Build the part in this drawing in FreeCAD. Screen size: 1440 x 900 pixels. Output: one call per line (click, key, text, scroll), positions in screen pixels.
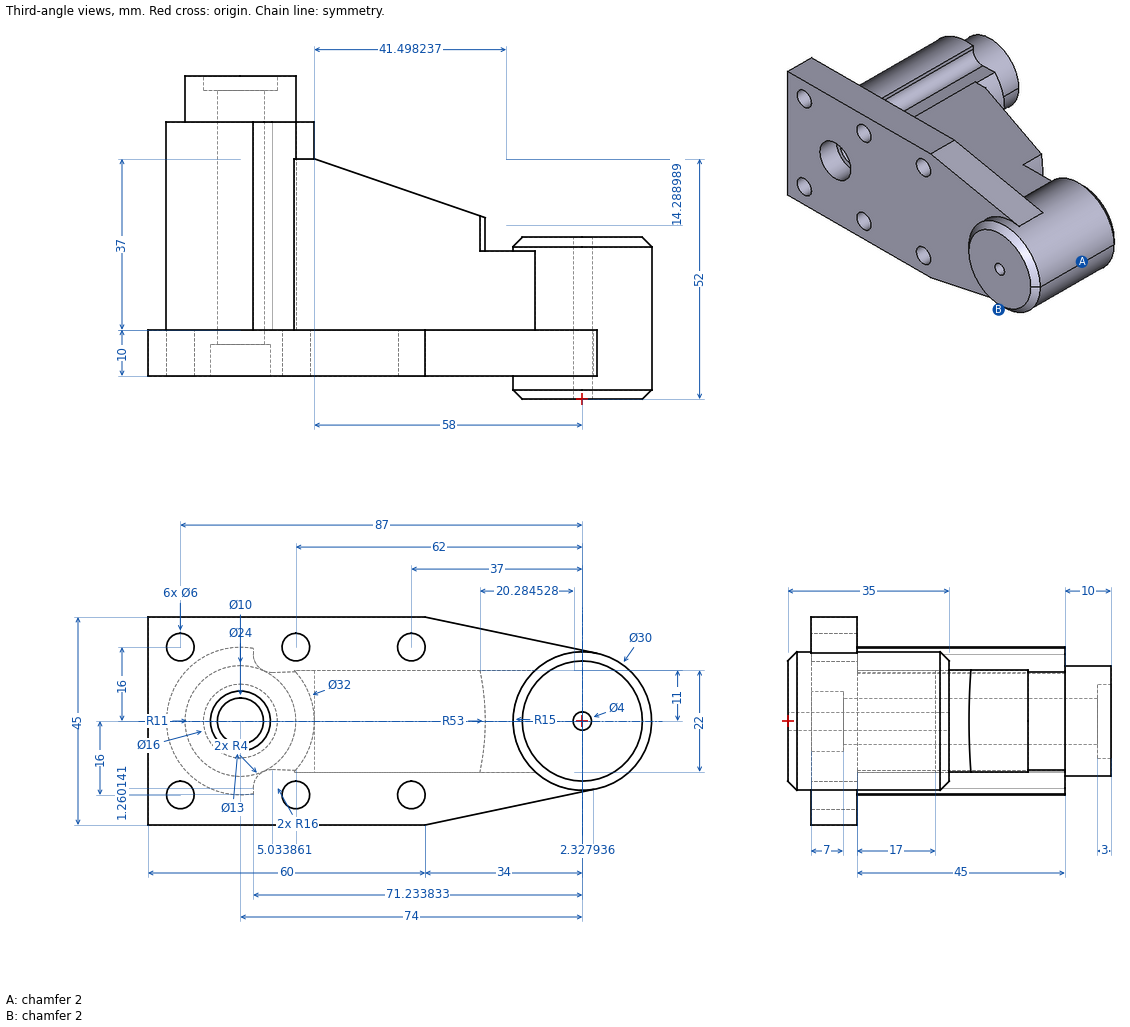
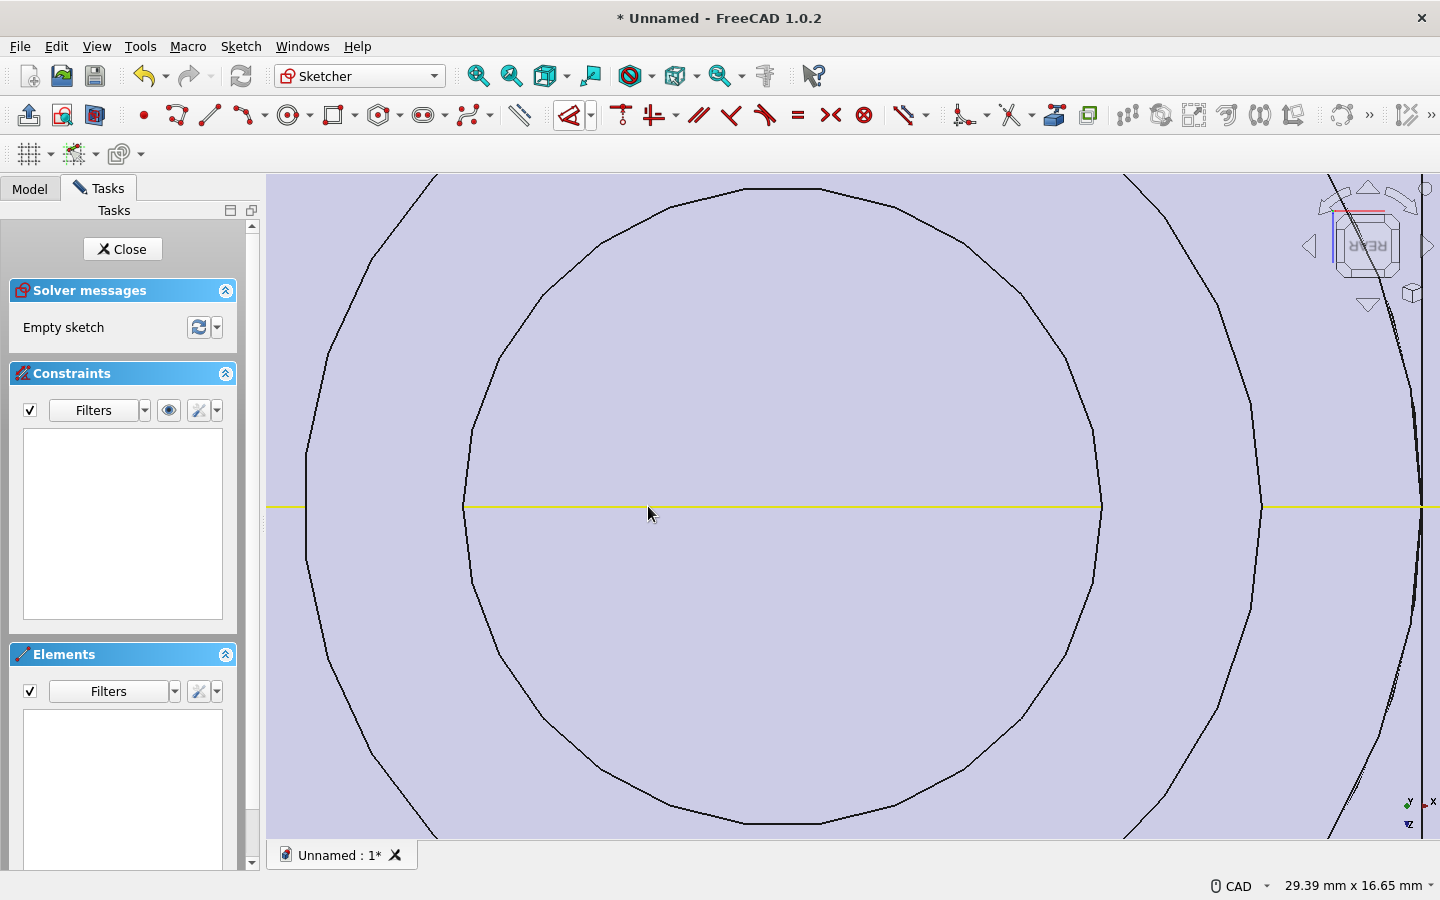
click(288, 116)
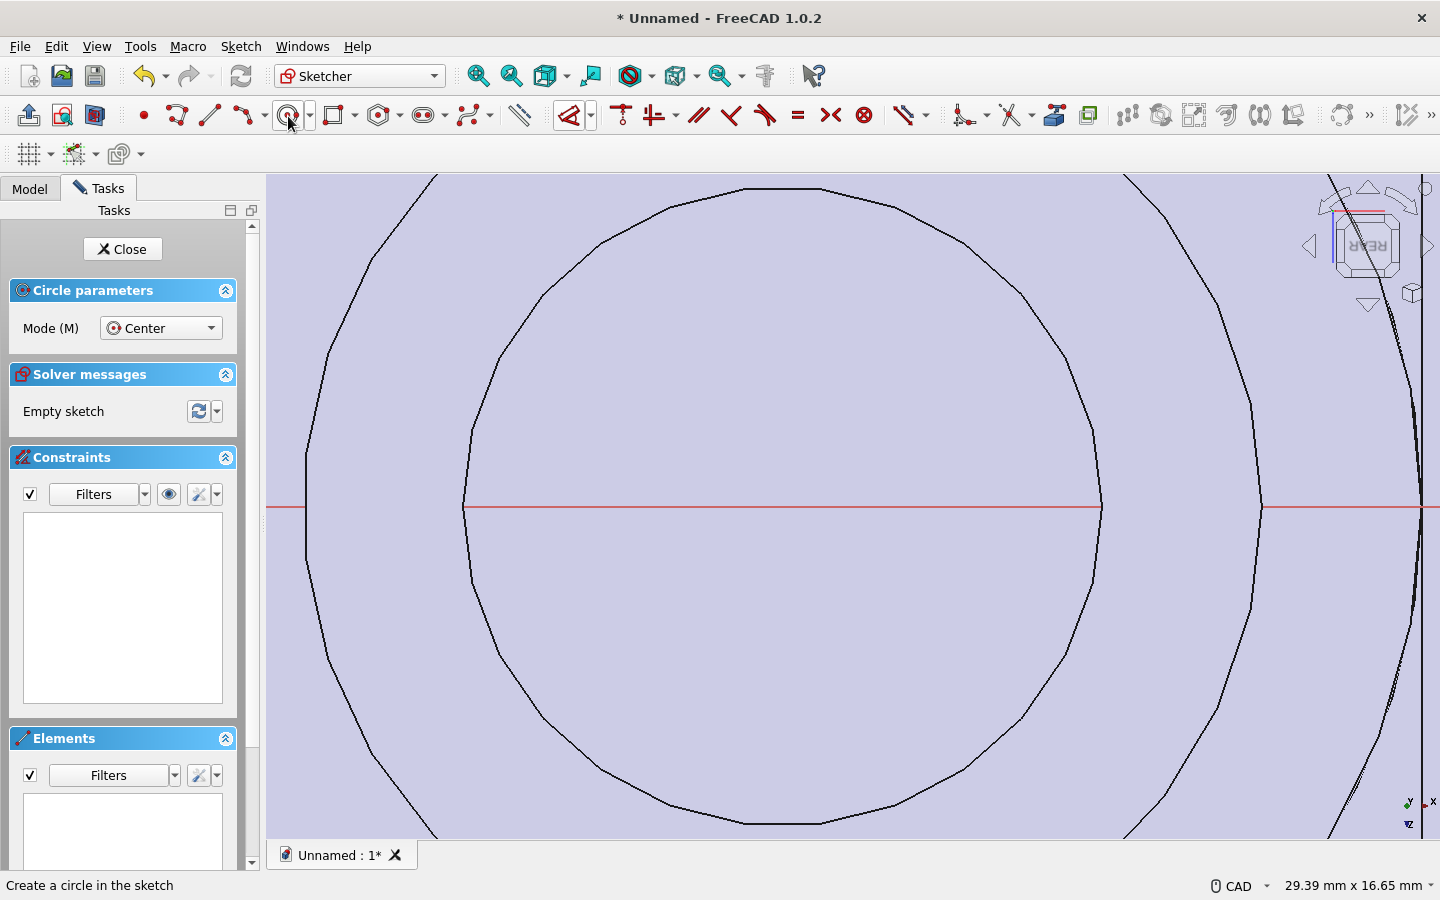
click(783, 506)
click(924, 365)
key(Escape)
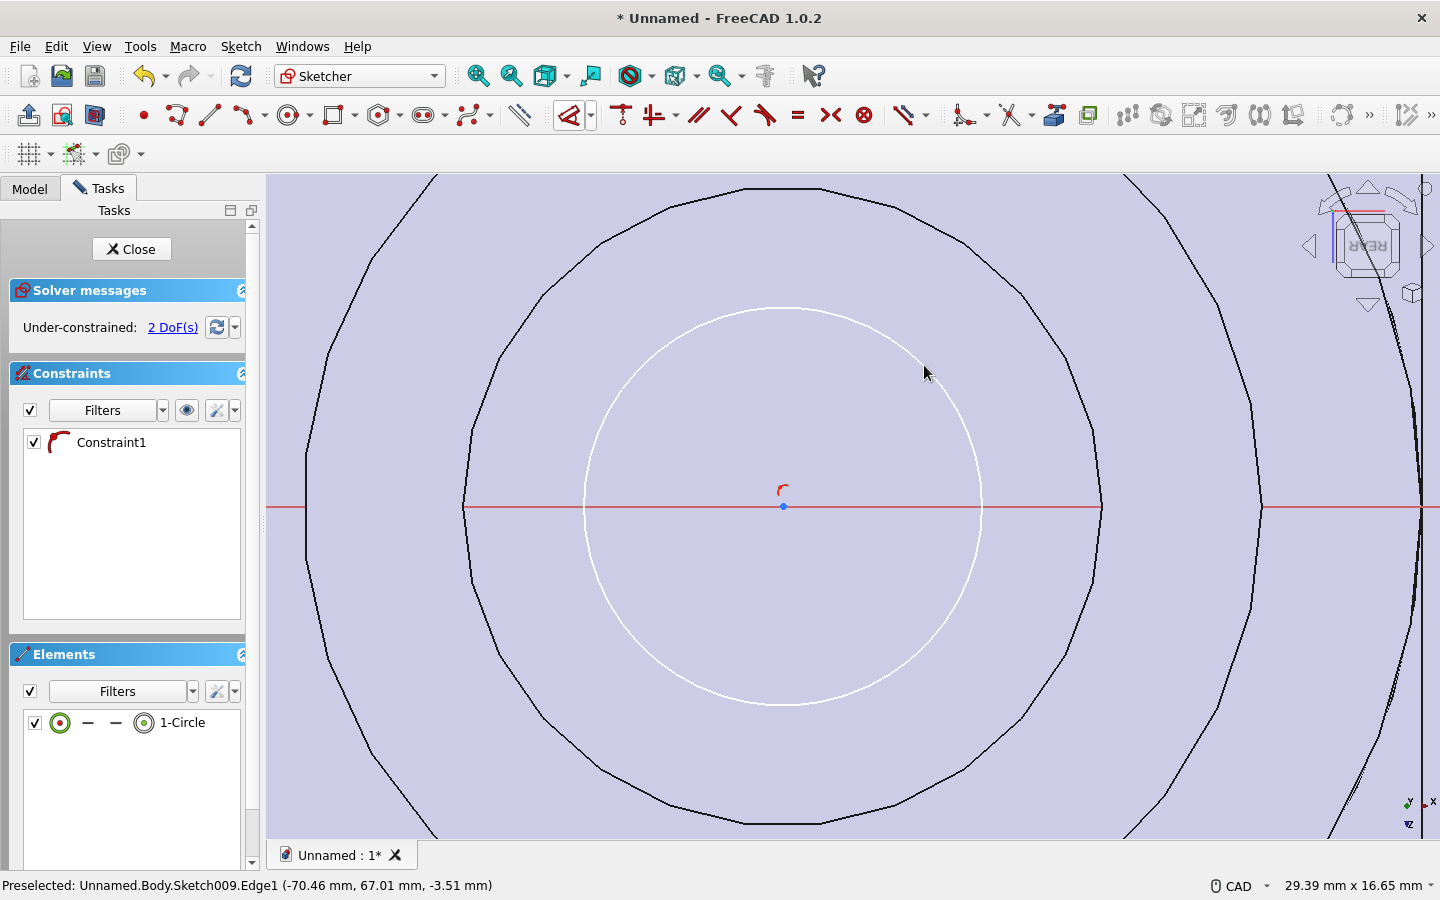
click(923, 365)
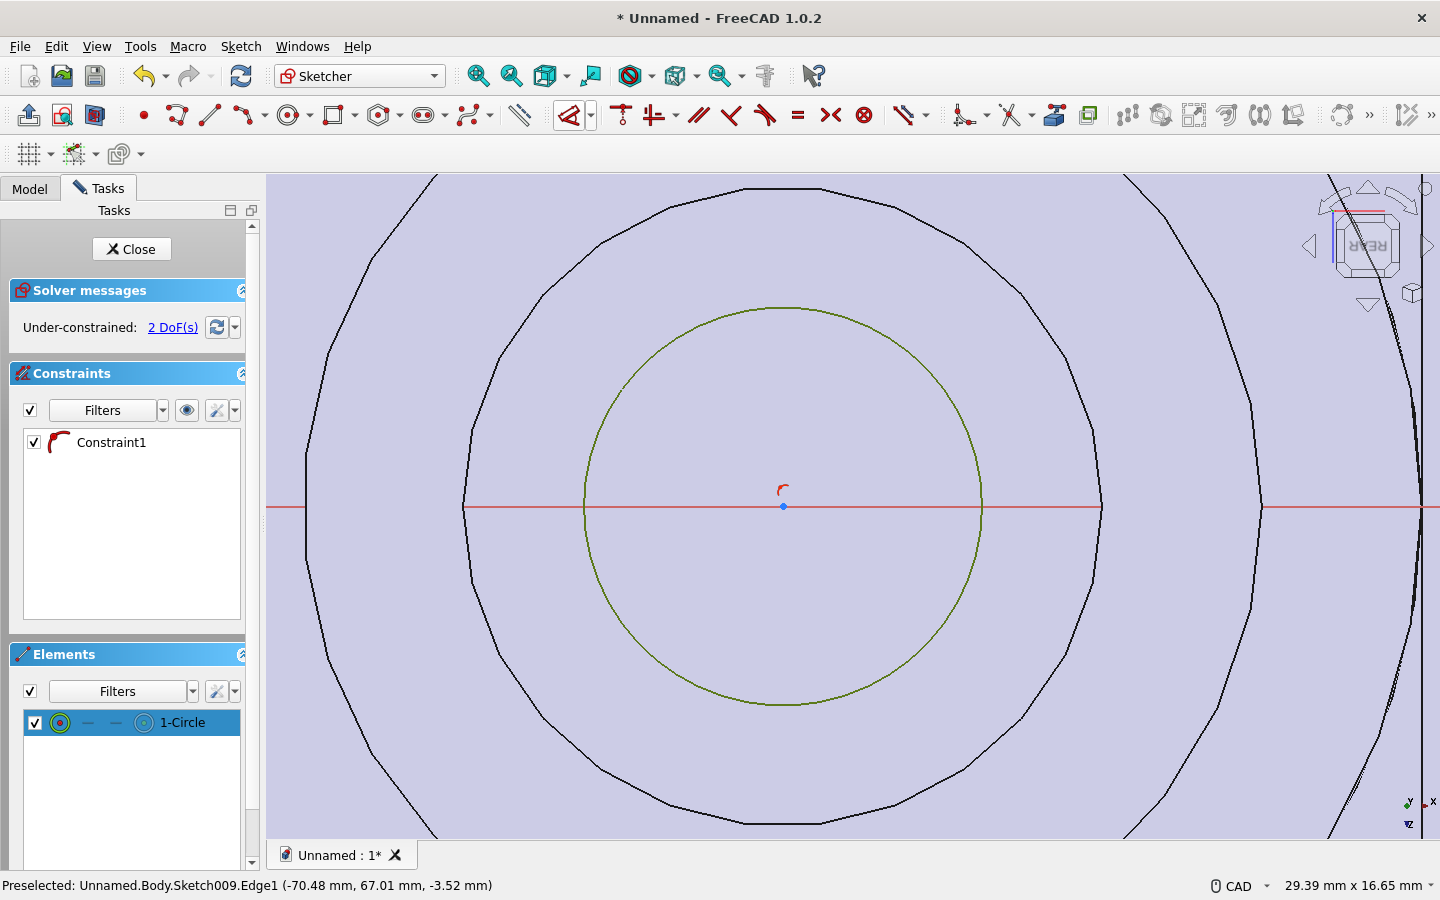
click(590, 116)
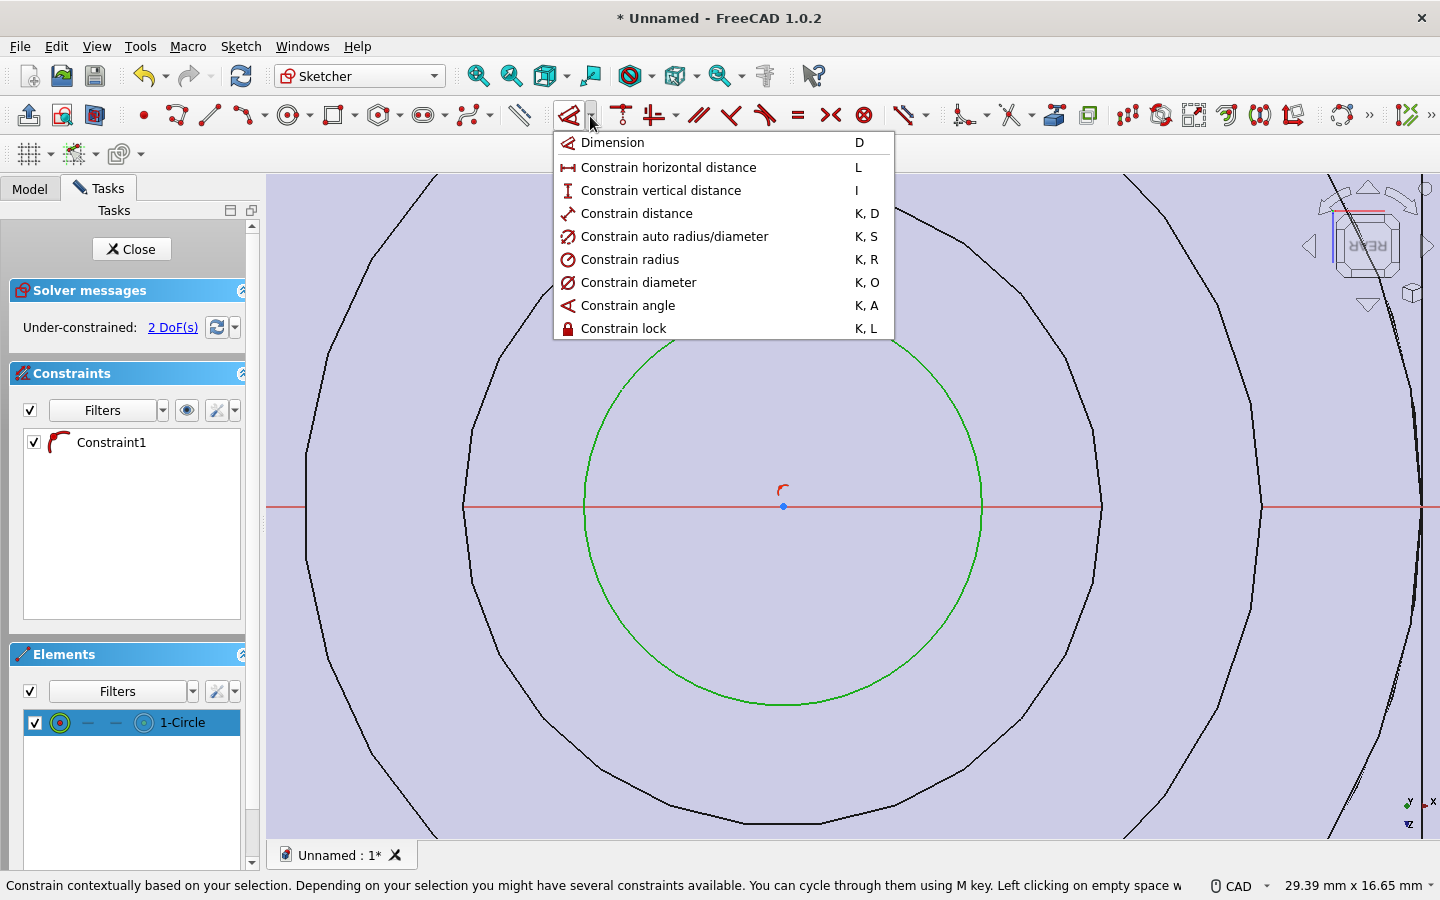
click(724, 282)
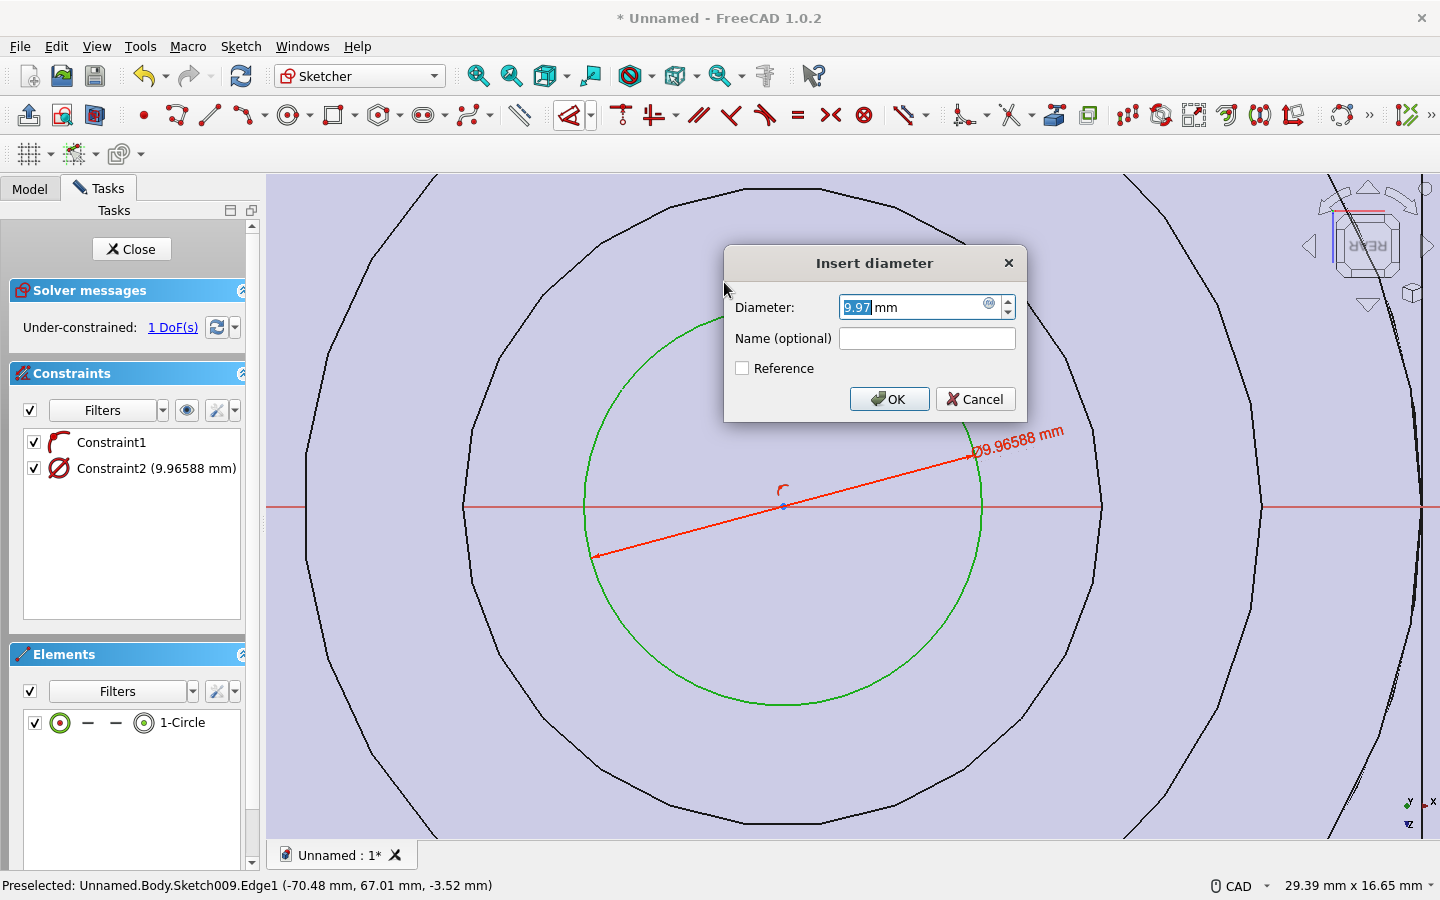
text(10)
key(Return)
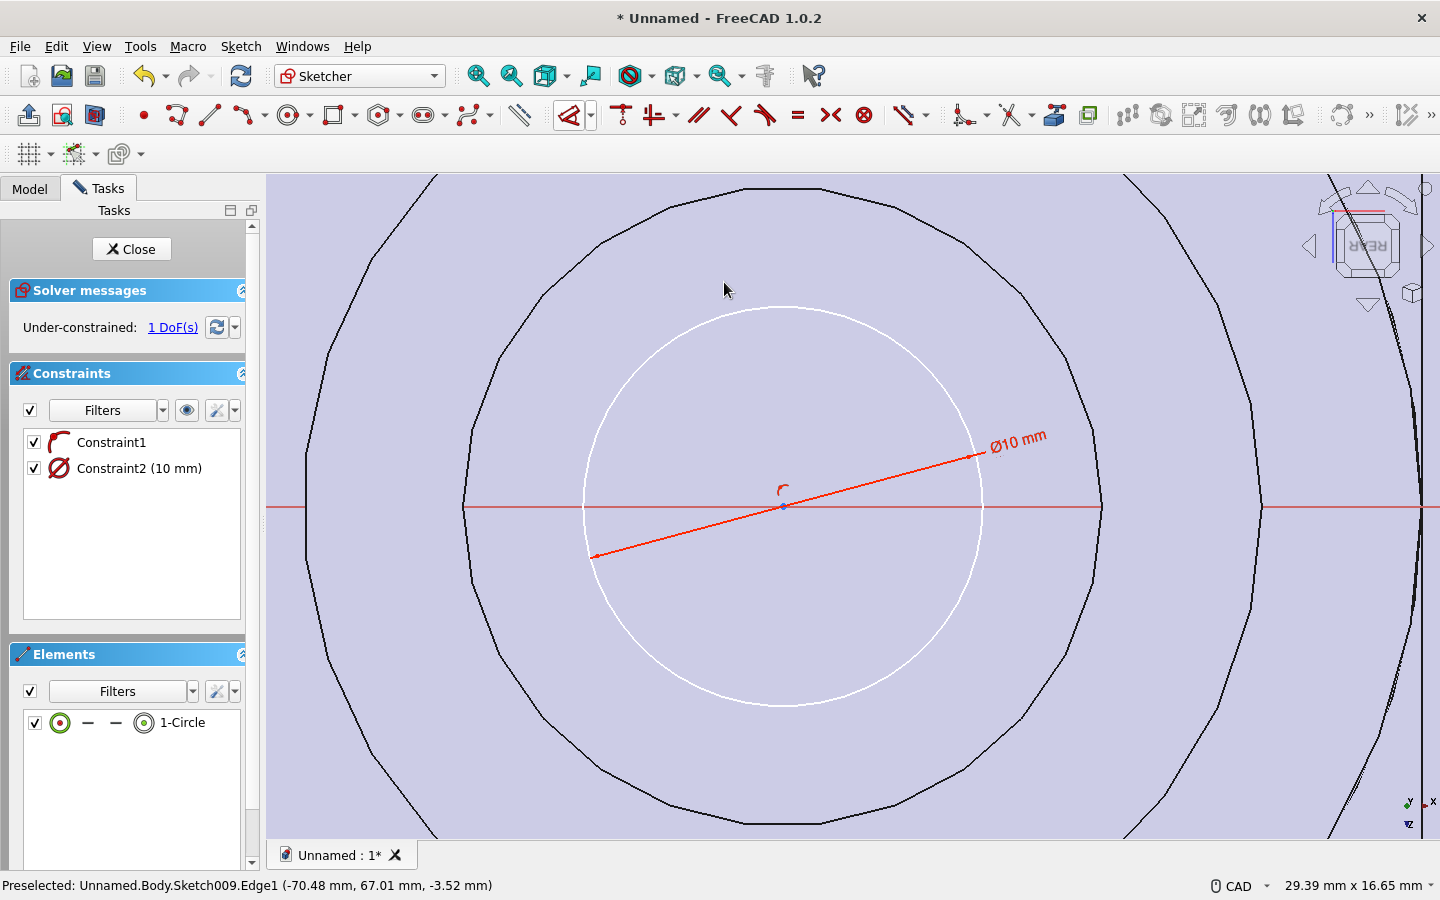
click(783, 506)